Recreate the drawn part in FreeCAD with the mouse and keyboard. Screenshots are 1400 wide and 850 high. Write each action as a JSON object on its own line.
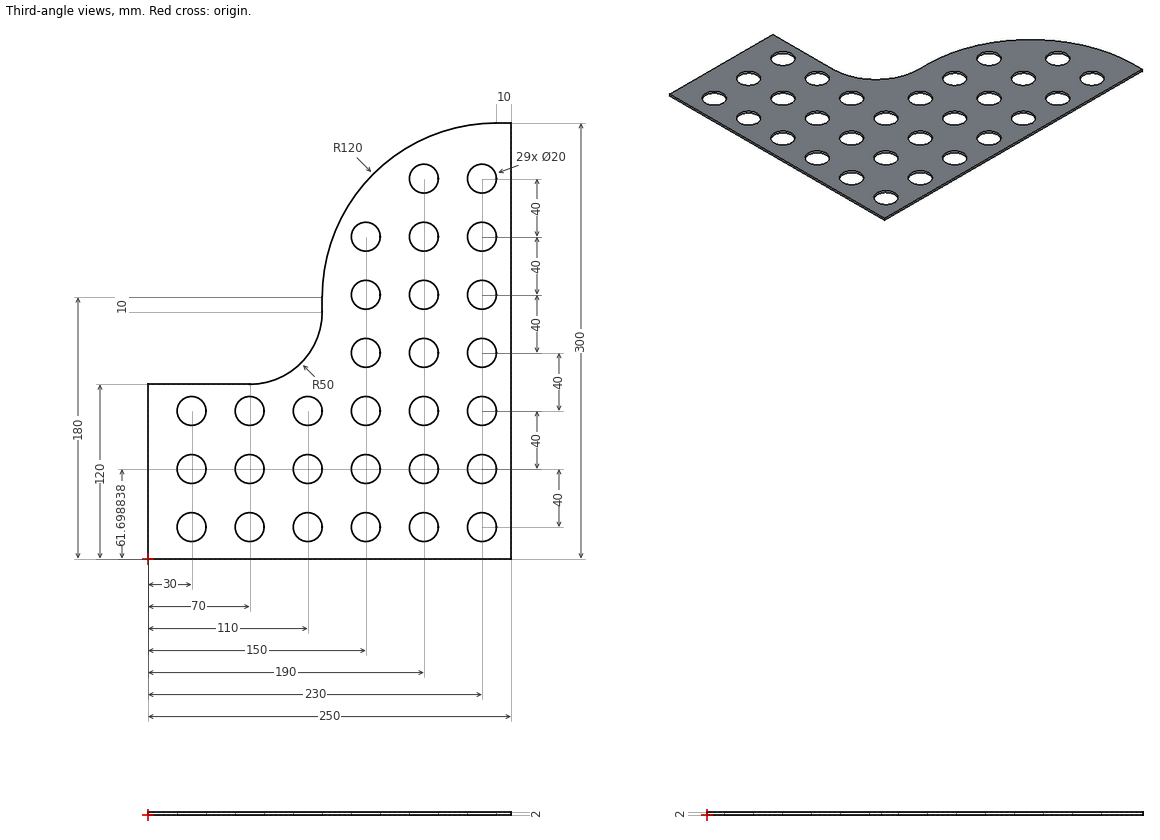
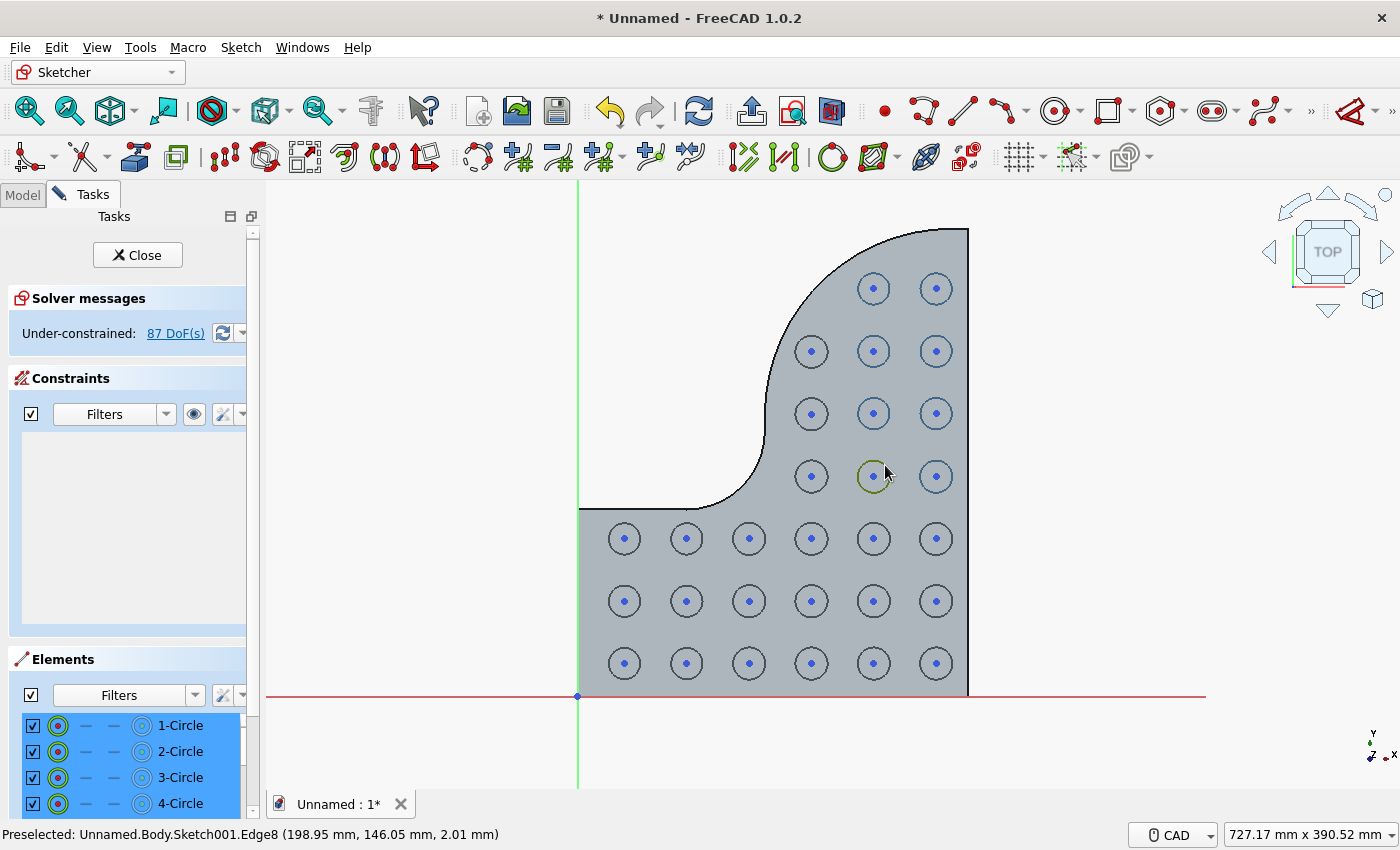
{"action": "left_click", "coordinate": [948, 528]}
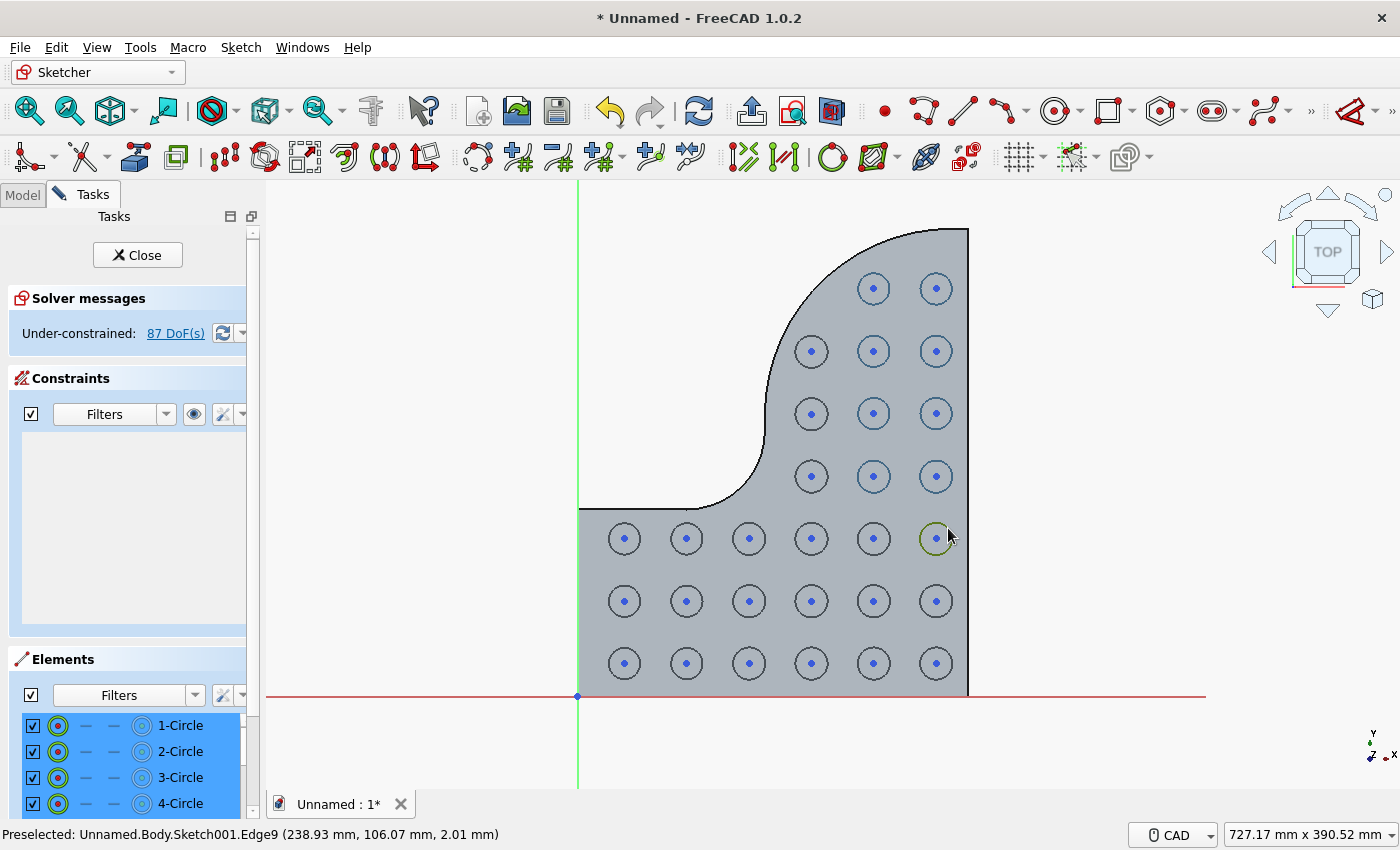
{"action": "left_click", "coordinate": [885, 528]}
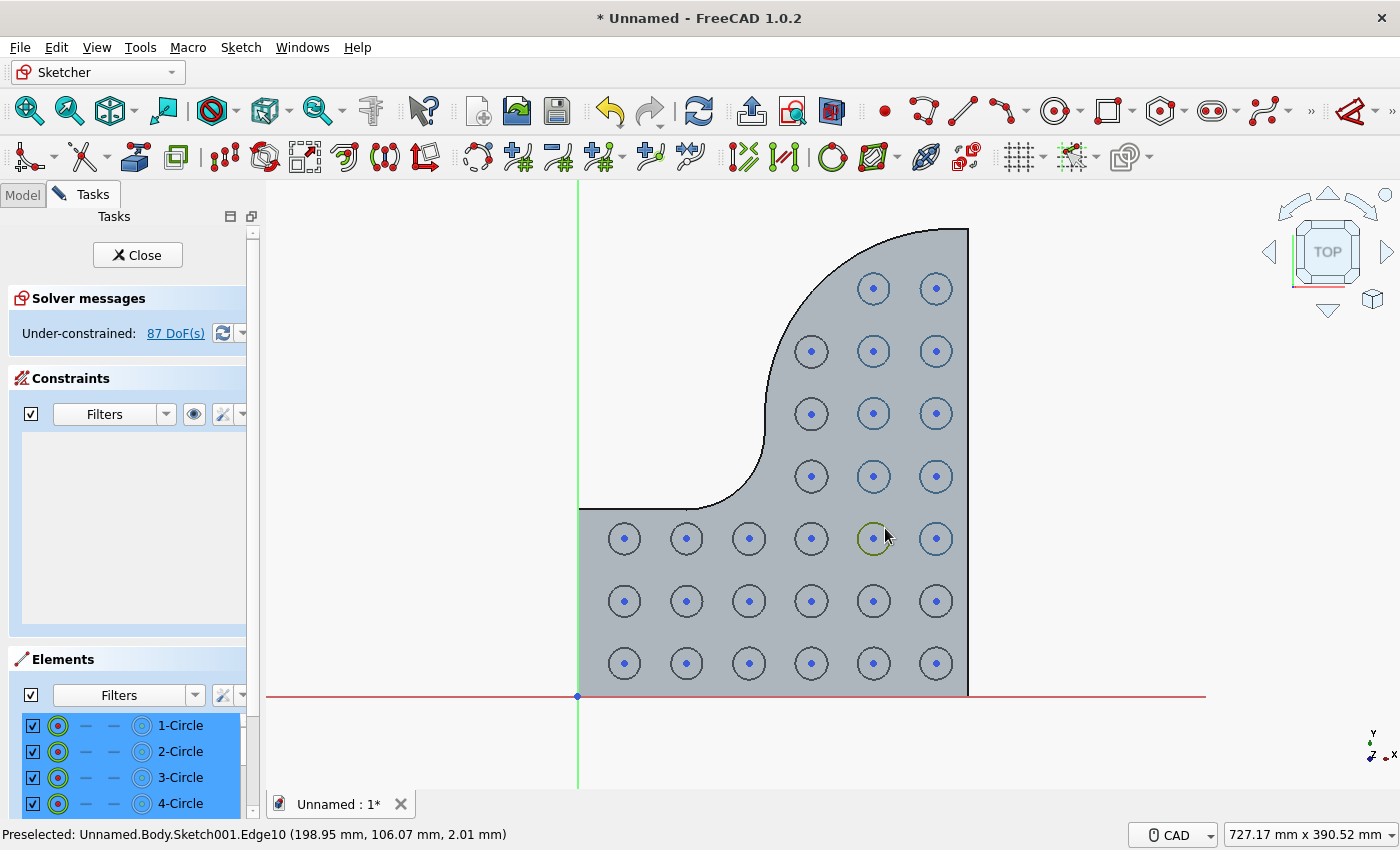
{"action": "left_click", "coordinate": [948, 590]}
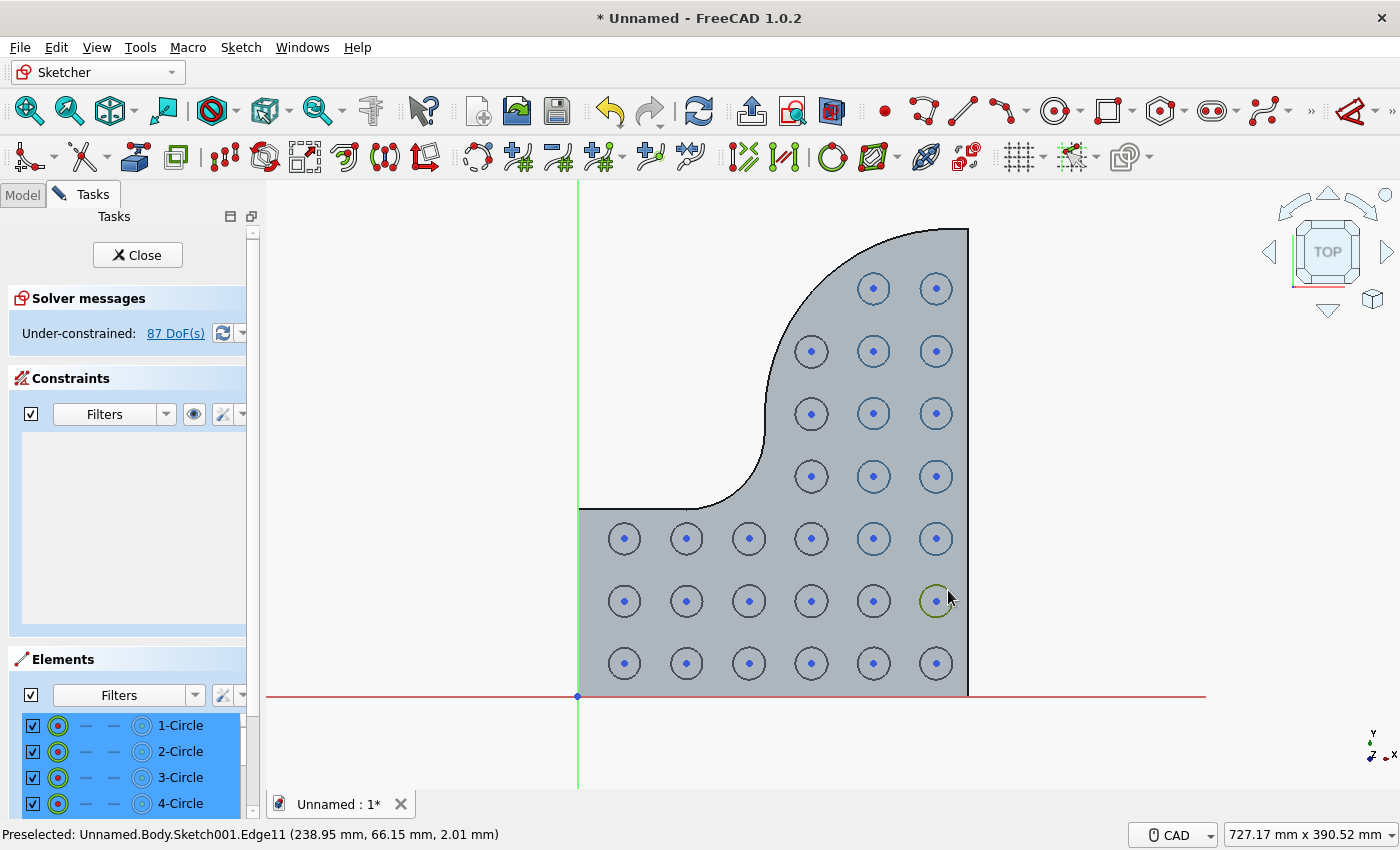
{"action": "left_click", "coordinate": [885, 590]}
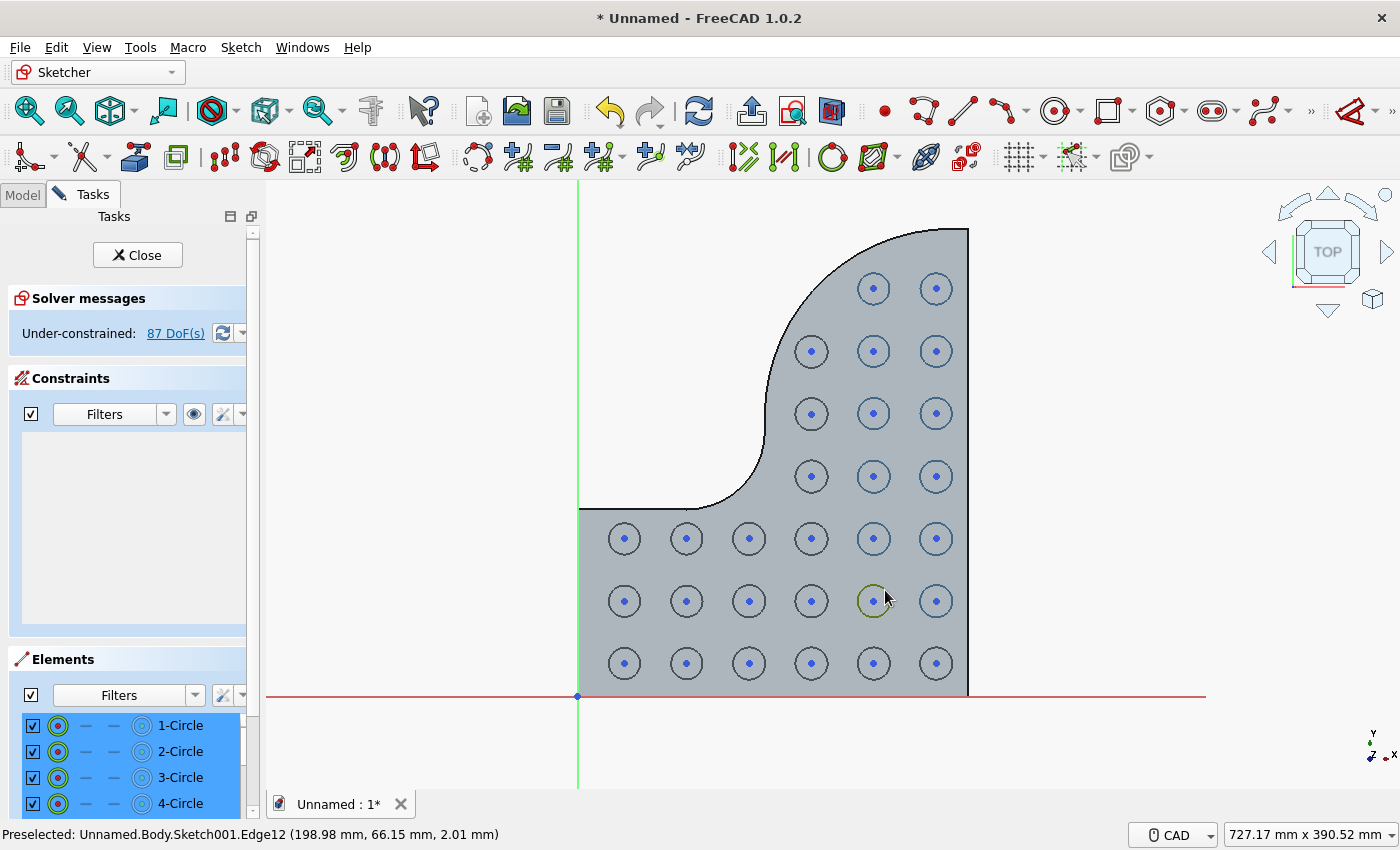
{"action": "left_click", "coordinate": [948, 652]}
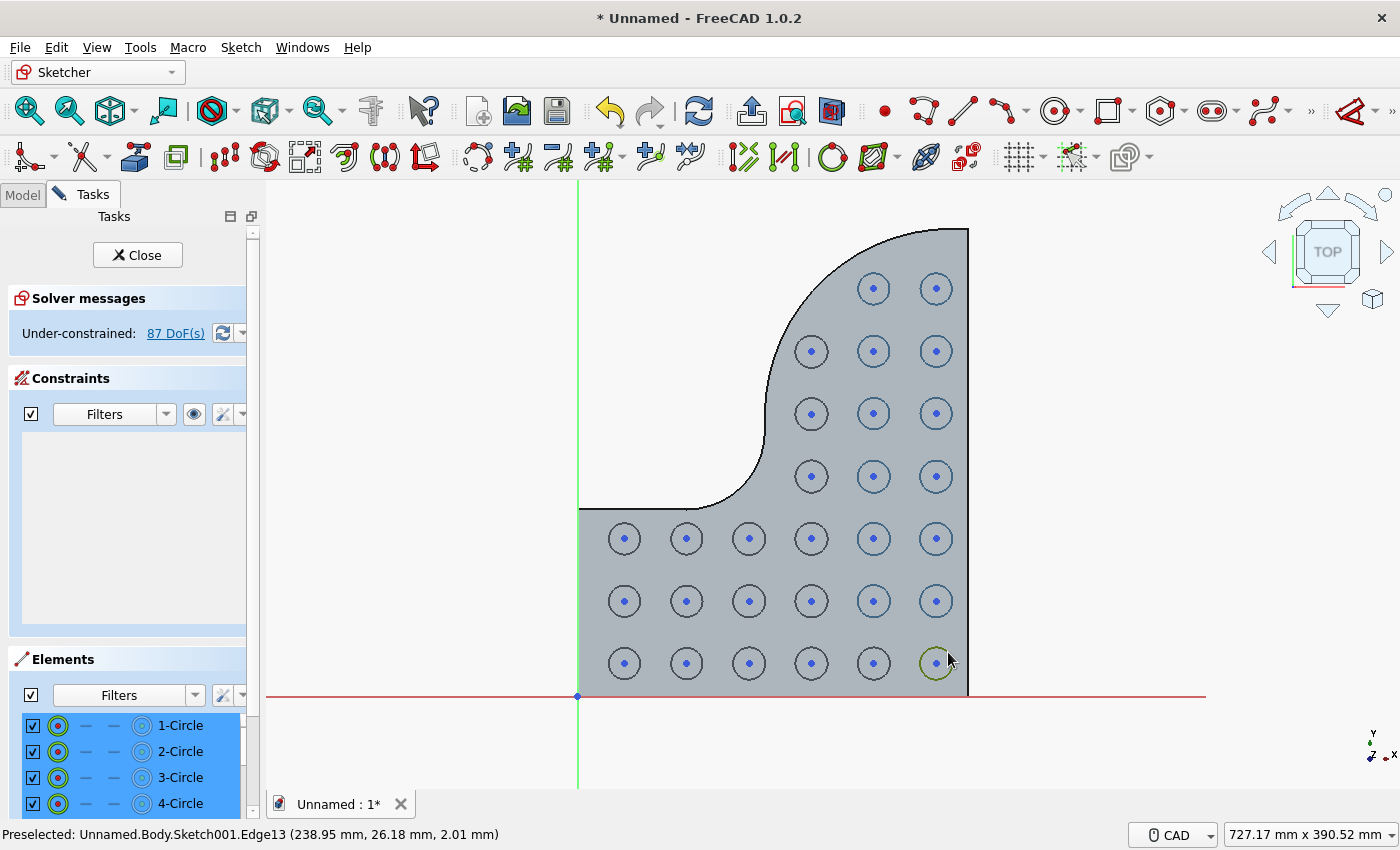
{"action": "left_click", "coordinate": [885, 652]}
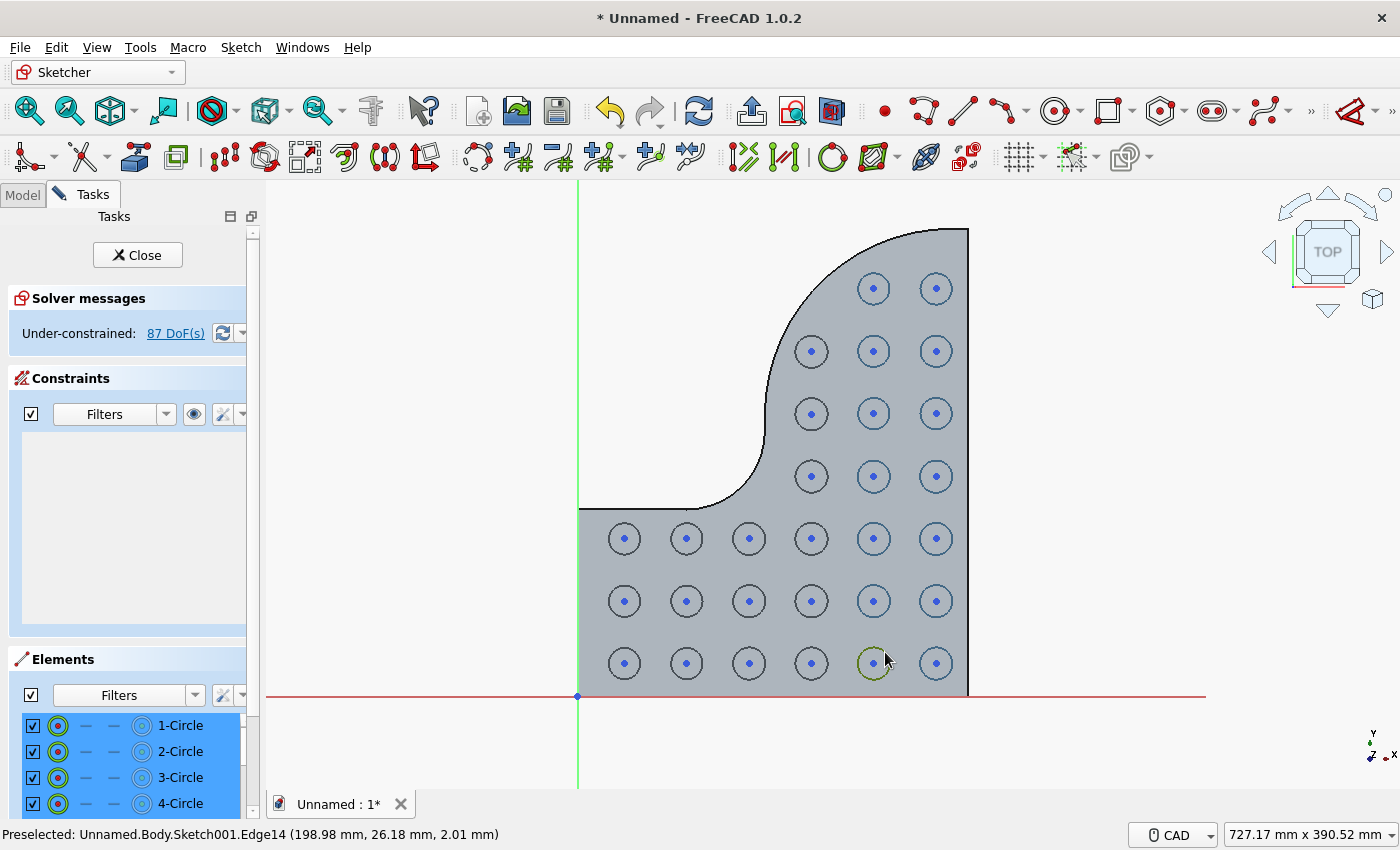
{"action": "left_click", "coordinate": [823, 340]}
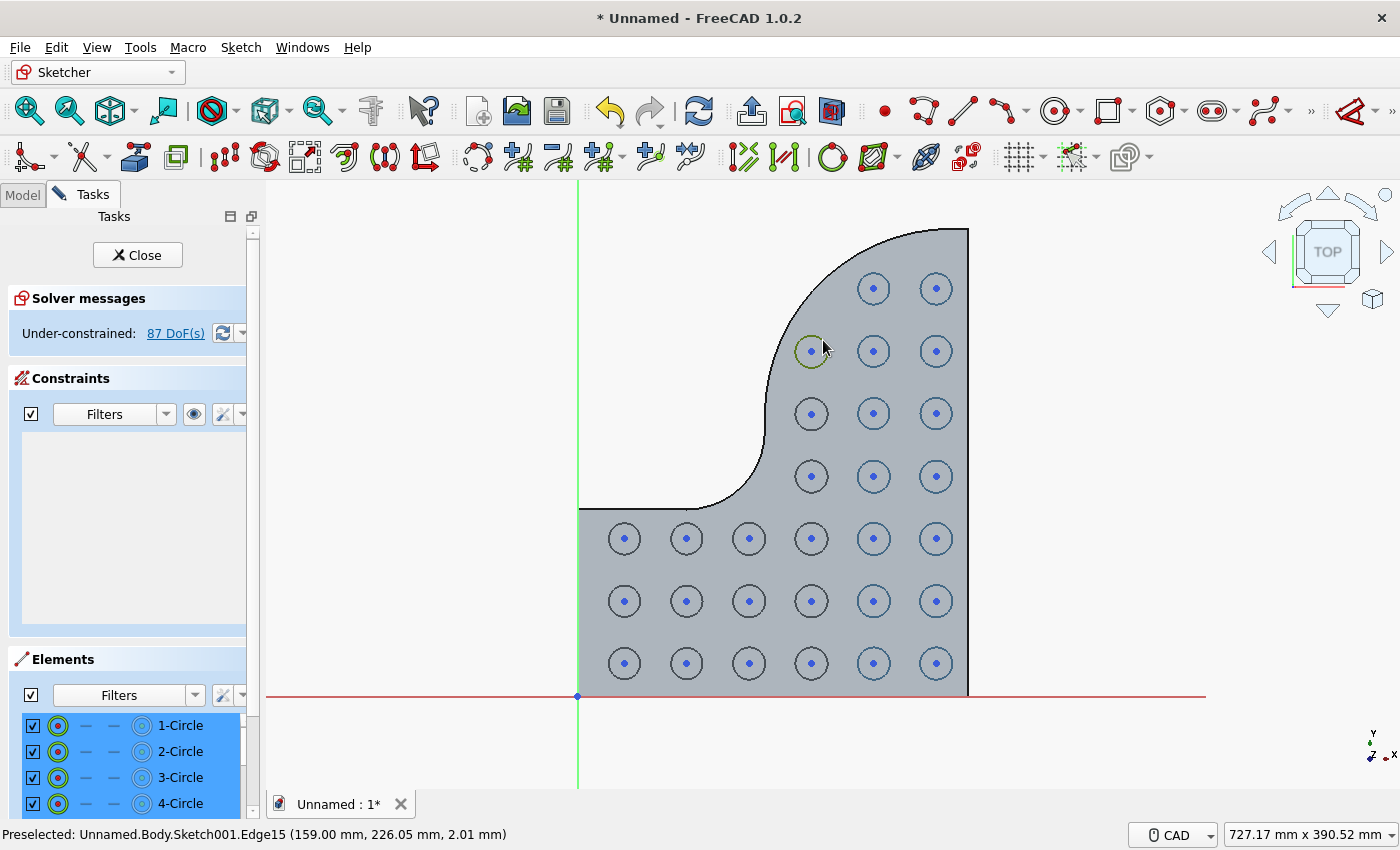
{"action": "left_click", "coordinate": [823, 403]}